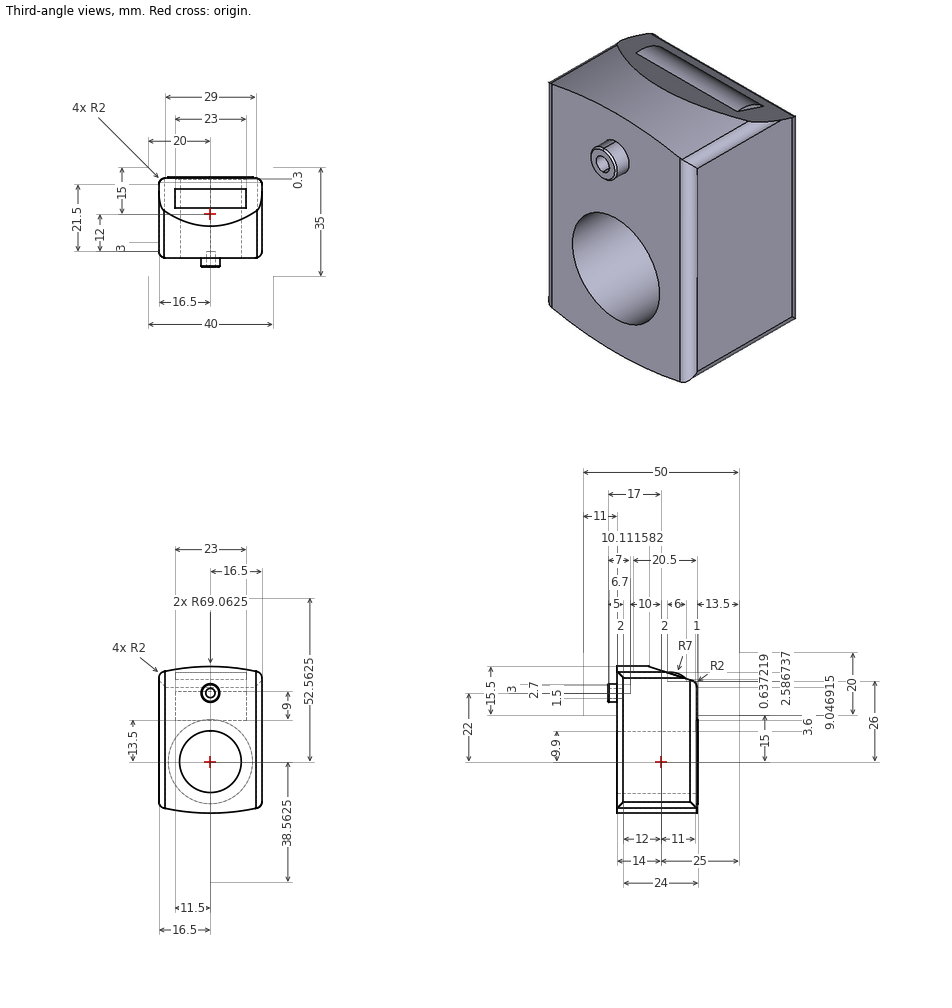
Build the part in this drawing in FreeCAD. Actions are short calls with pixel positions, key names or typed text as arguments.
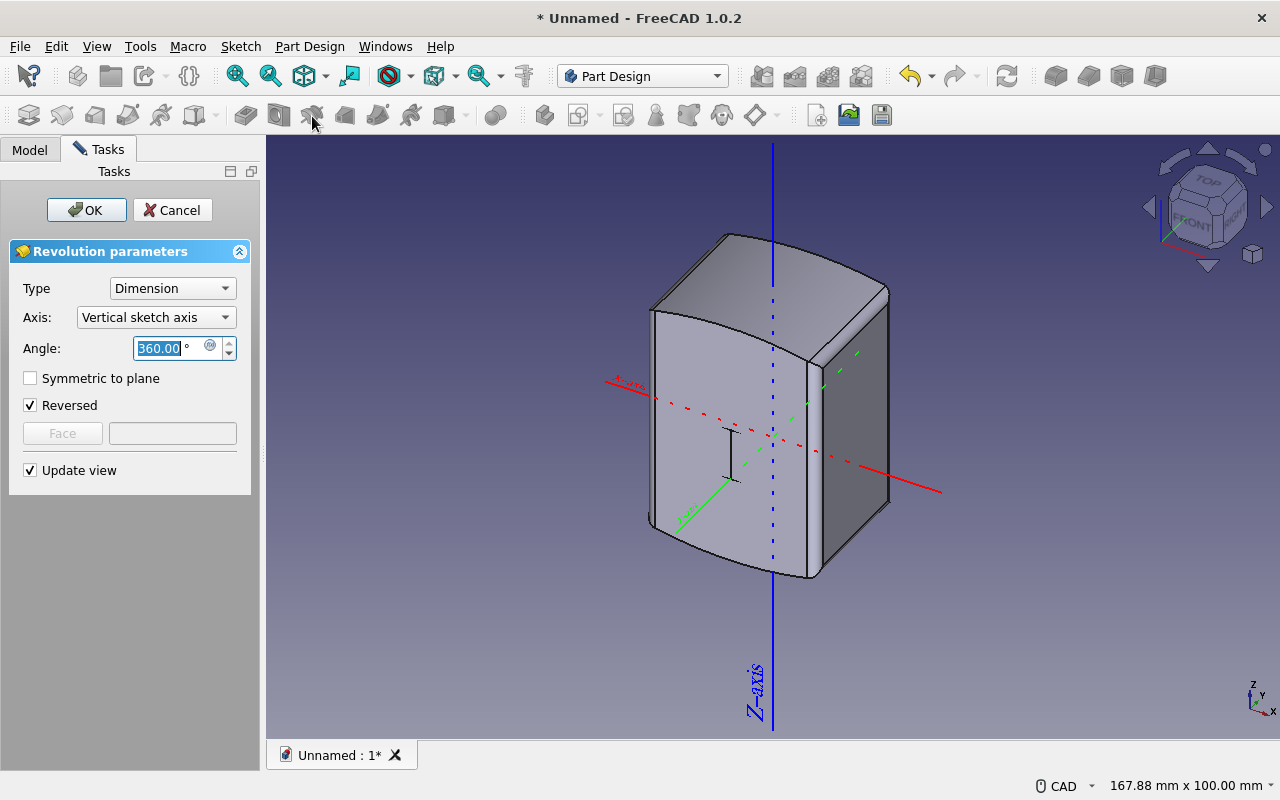
click(157, 318)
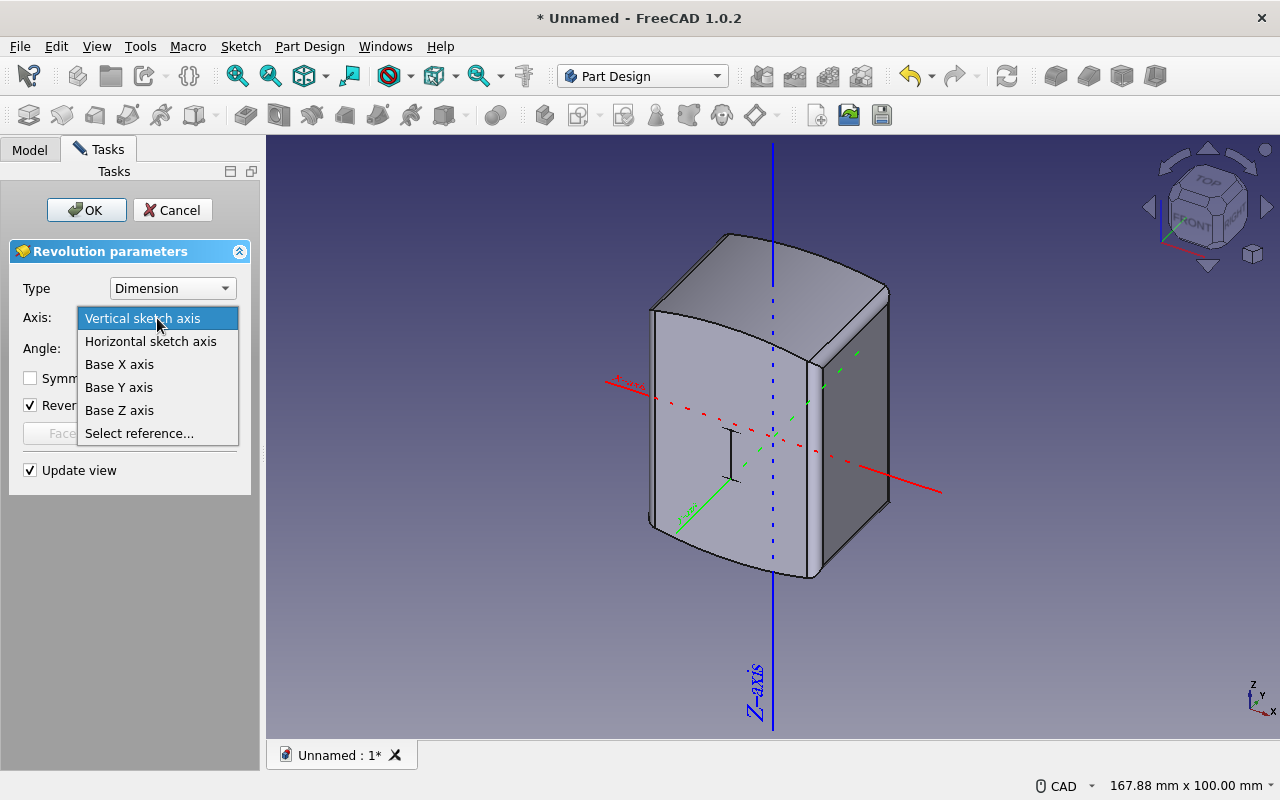
click(156, 342)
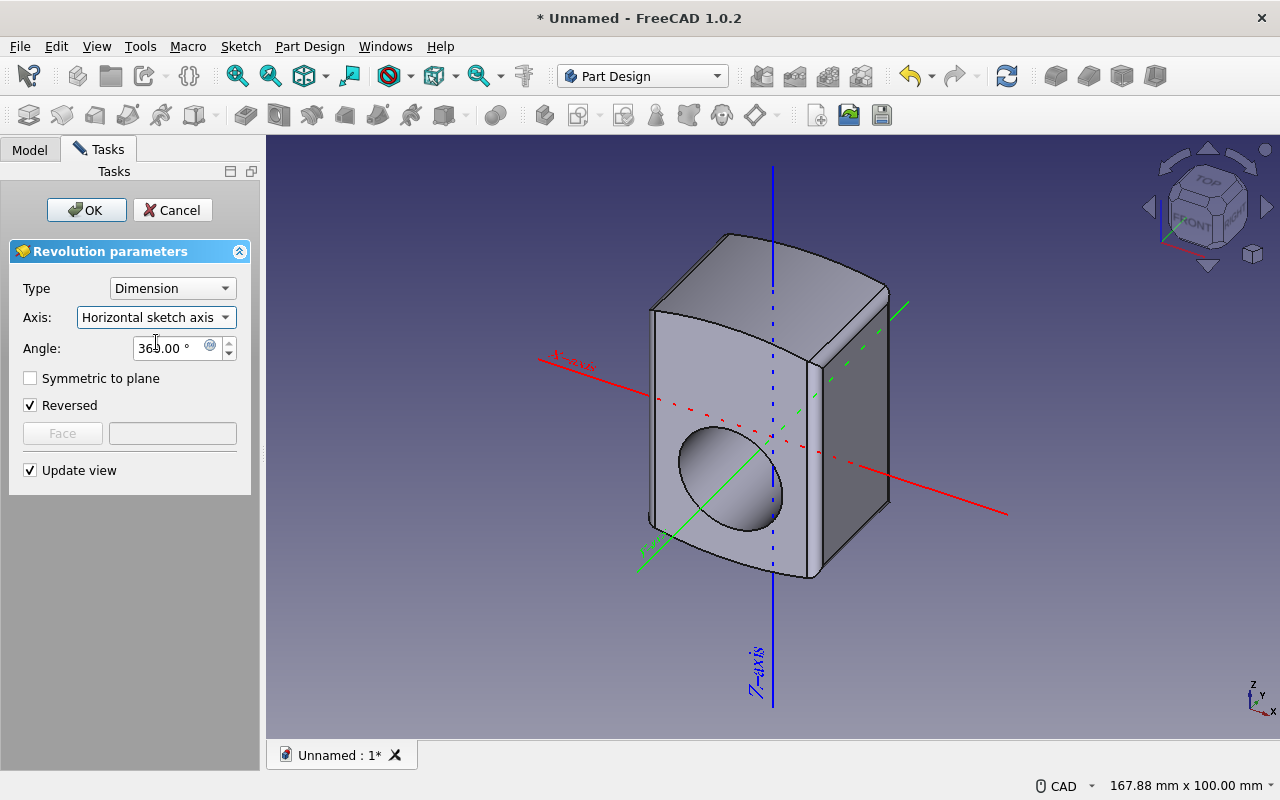
click(87, 210)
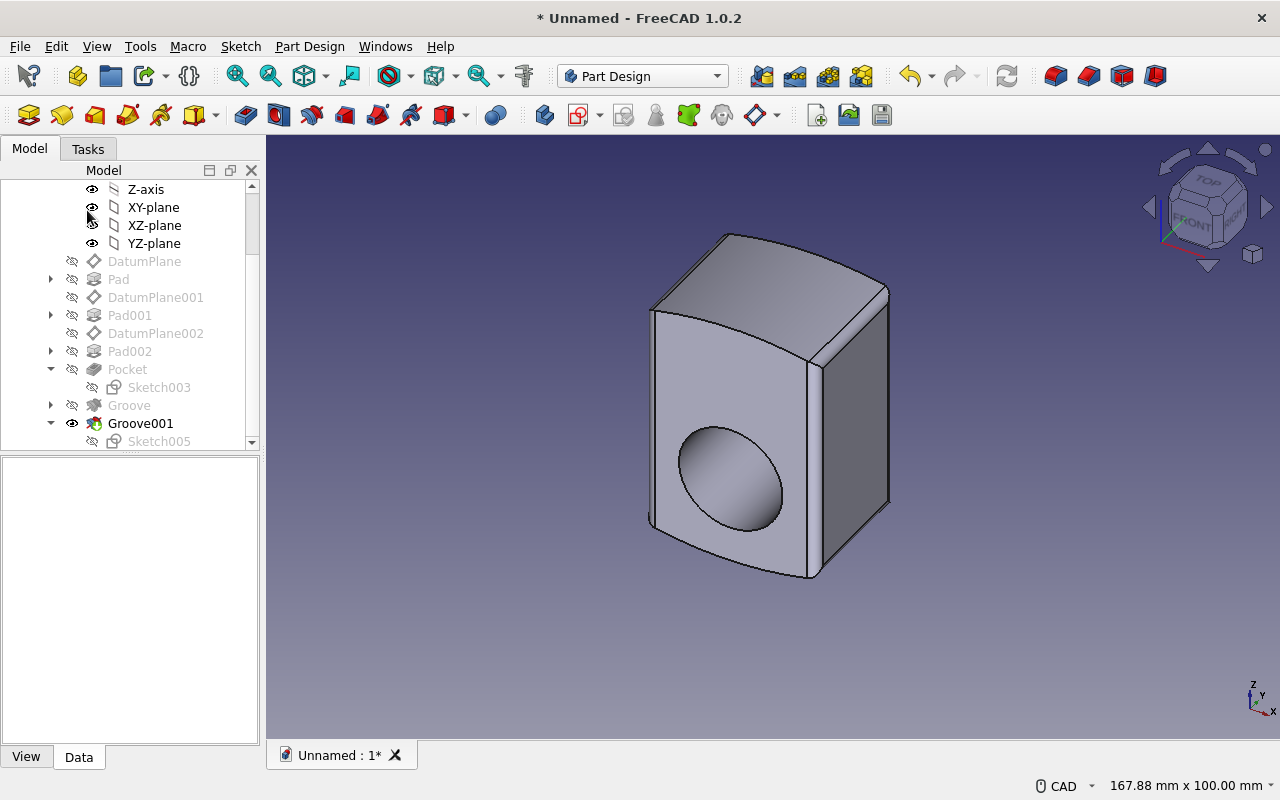
click(578, 116)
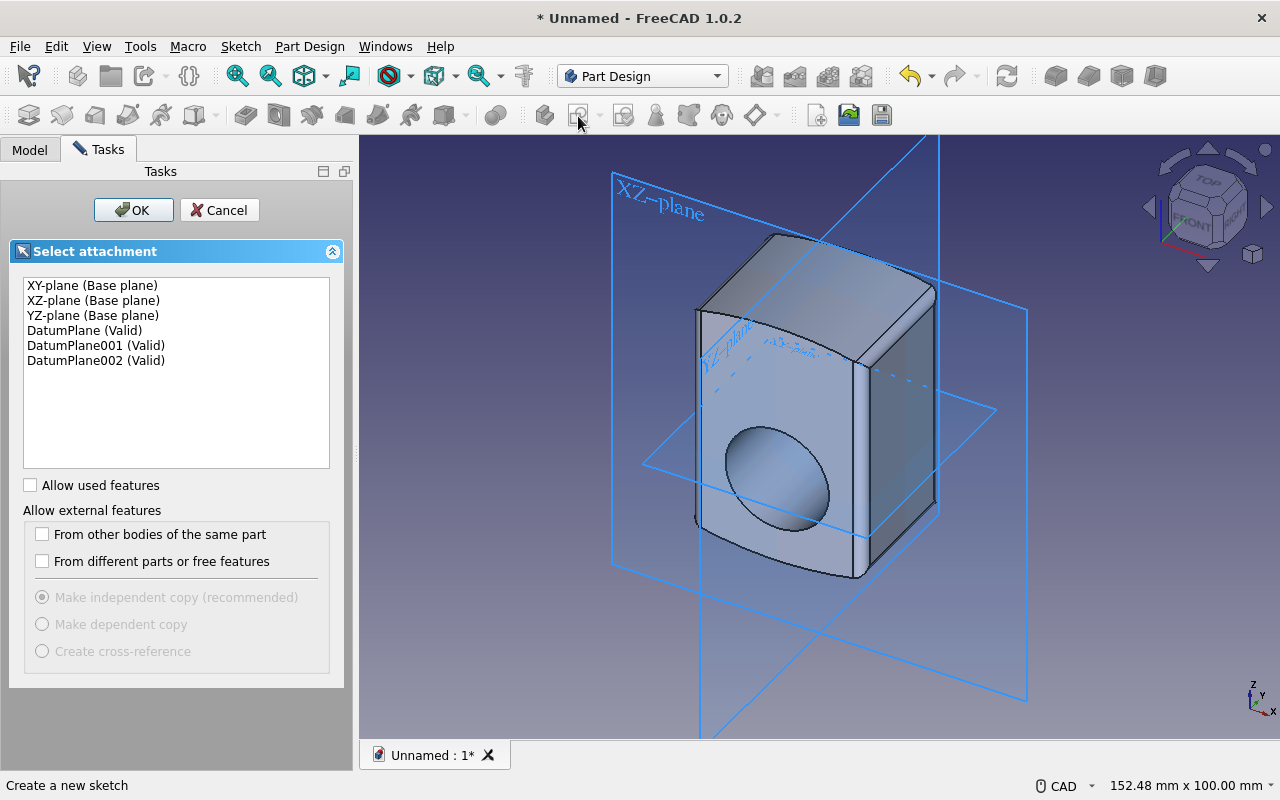
click(84, 316)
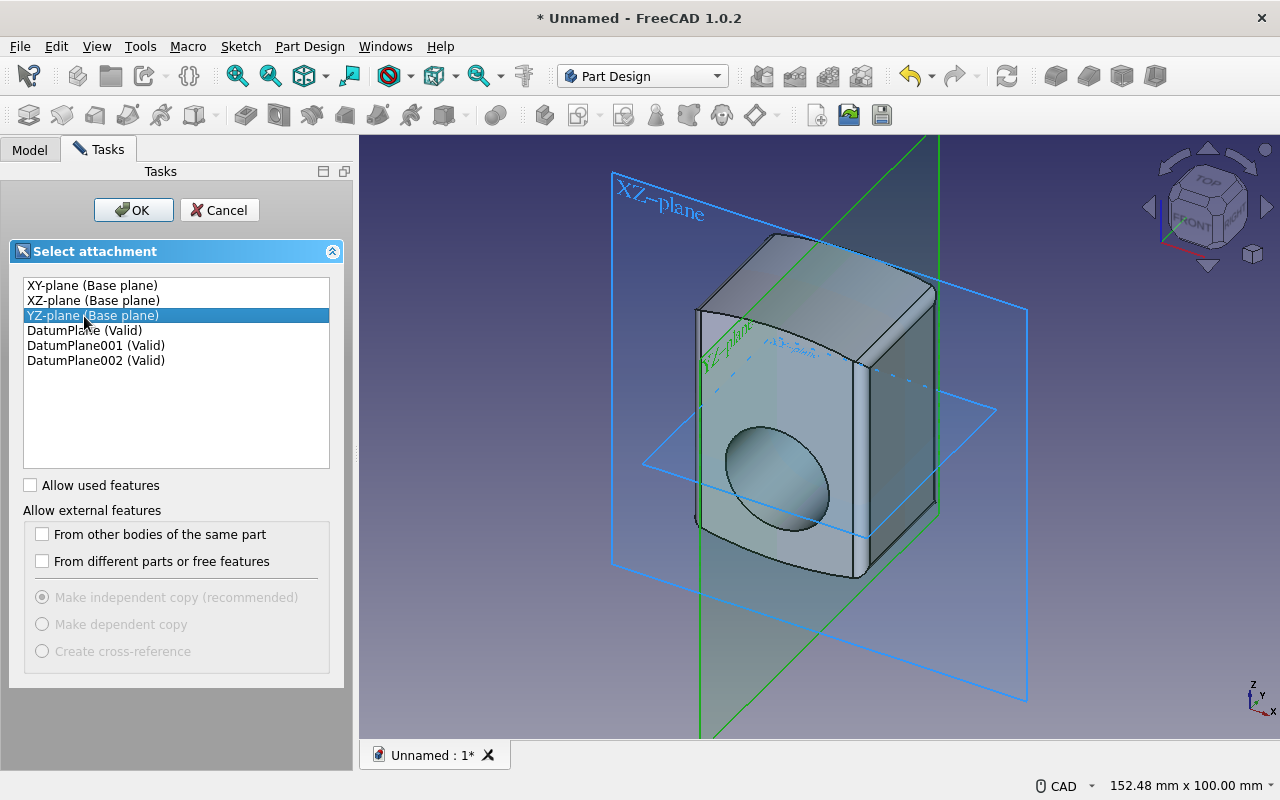
click(134, 210)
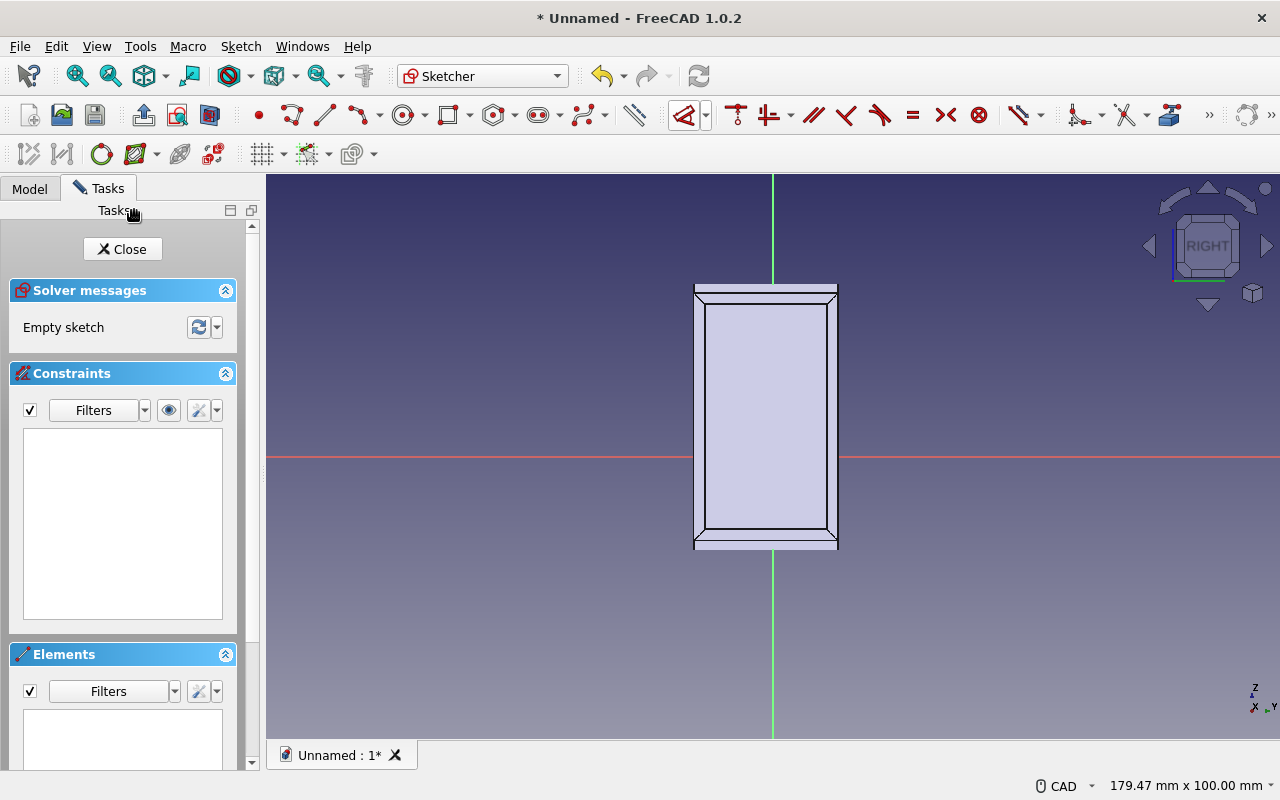
click(210, 116)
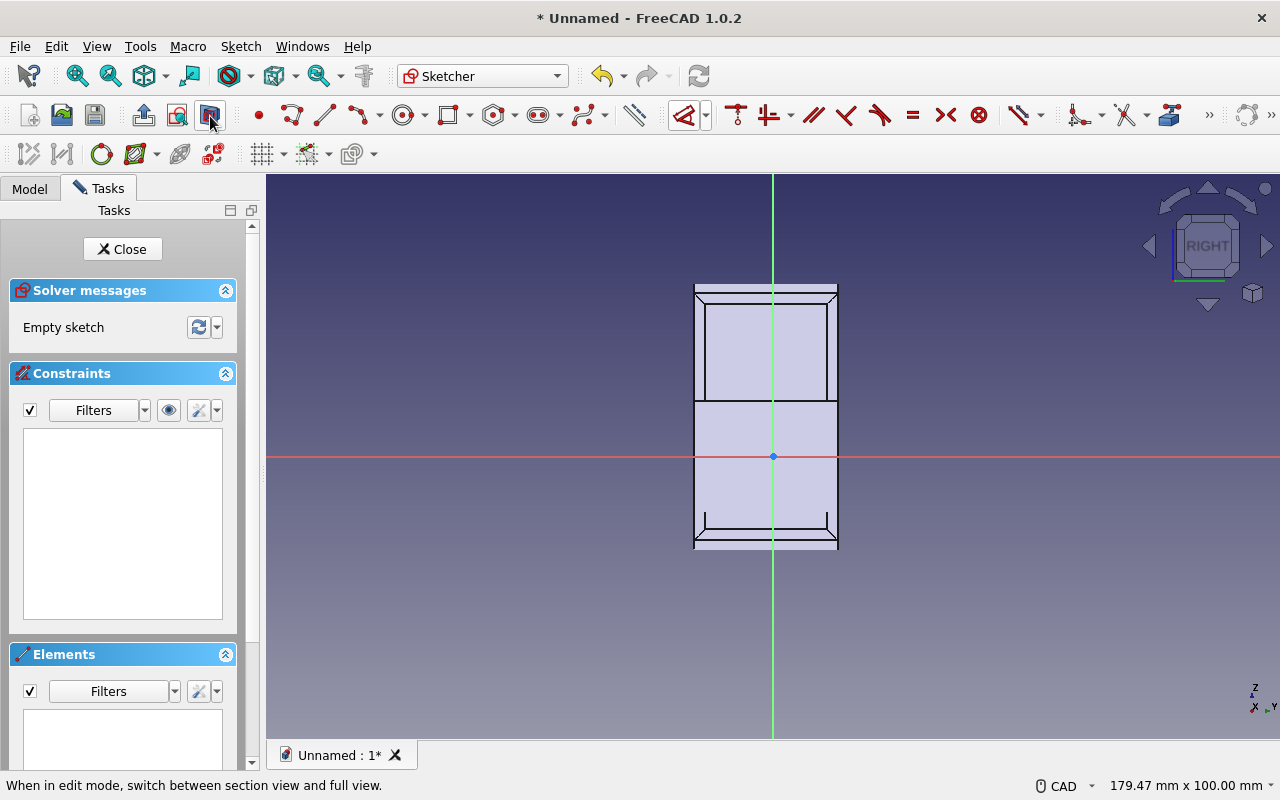
scroll(856, 237, up, 3)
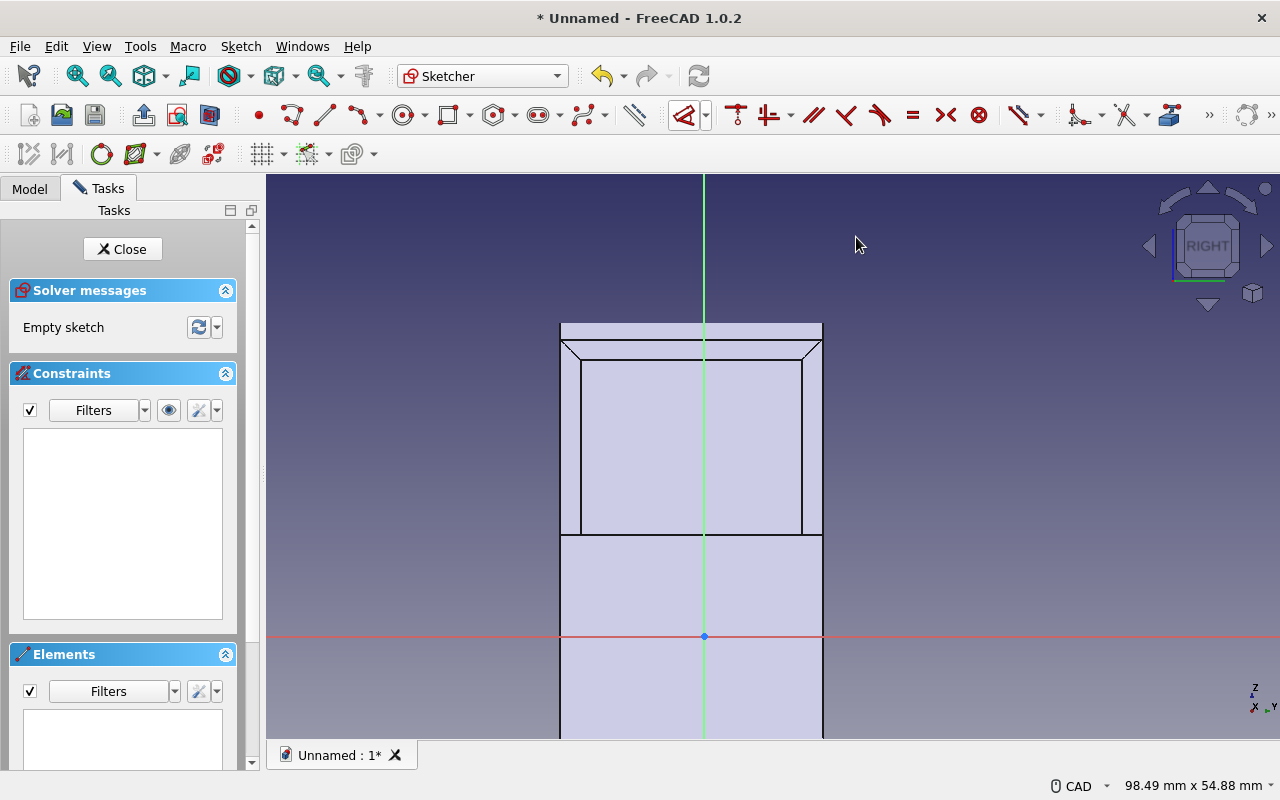
click(292, 116)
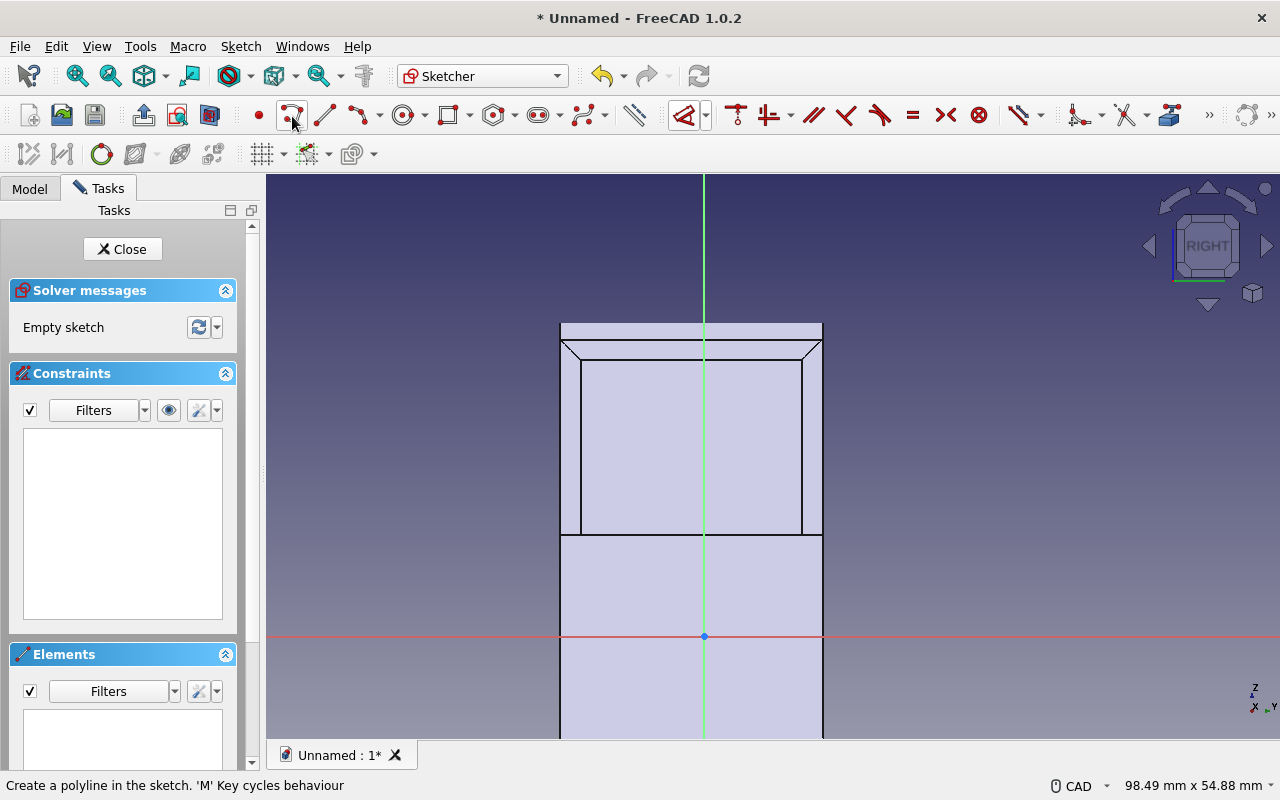
click(823, 389)
click(823, 482)
click(962, 482)
click(962, 277)
click(447, 277)
click(447, 482)
click(560, 482)
click(560, 323)
click(664, 323)
click(808, 370)
right_click(808, 370)